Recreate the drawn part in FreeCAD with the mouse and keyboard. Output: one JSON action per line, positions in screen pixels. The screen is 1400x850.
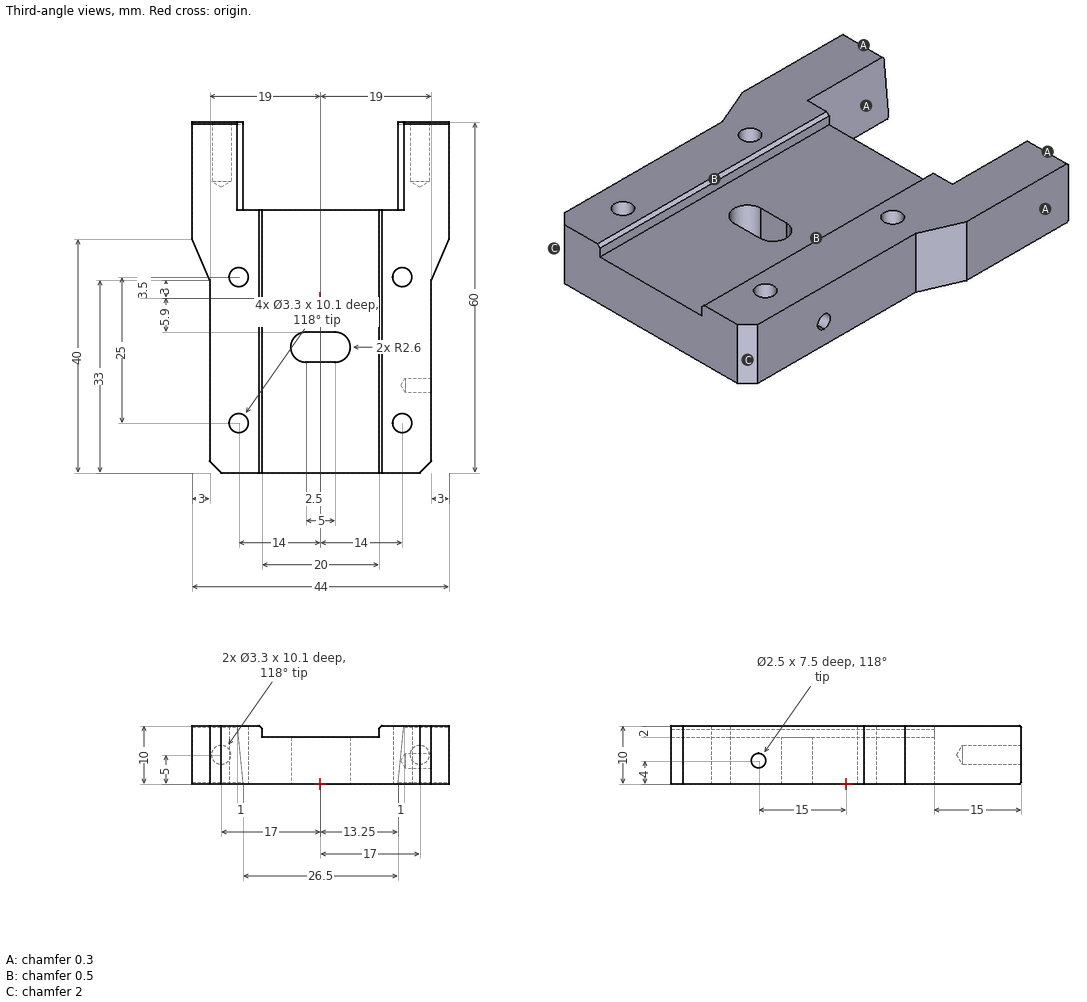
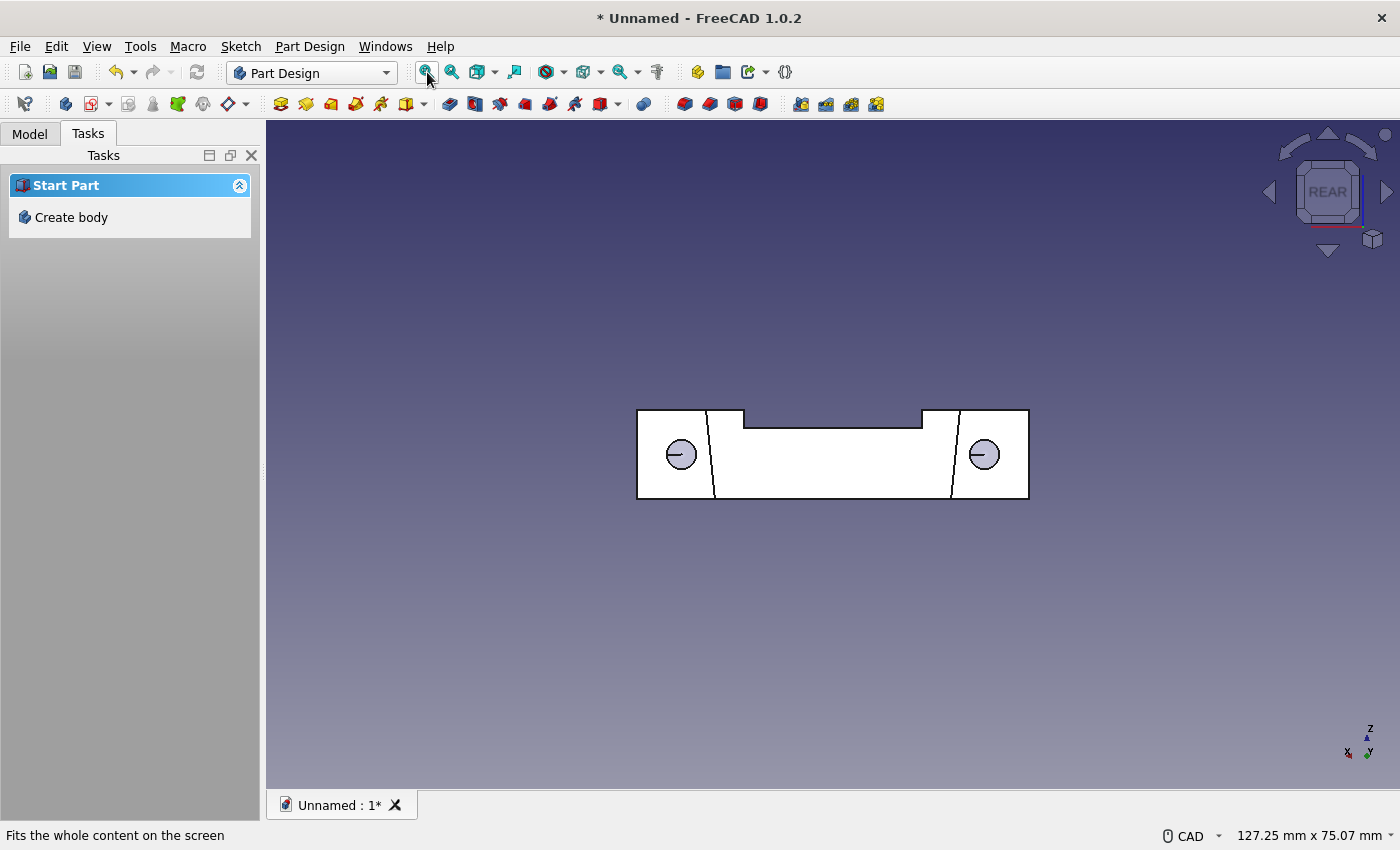
{"action": "key", "text": "0"}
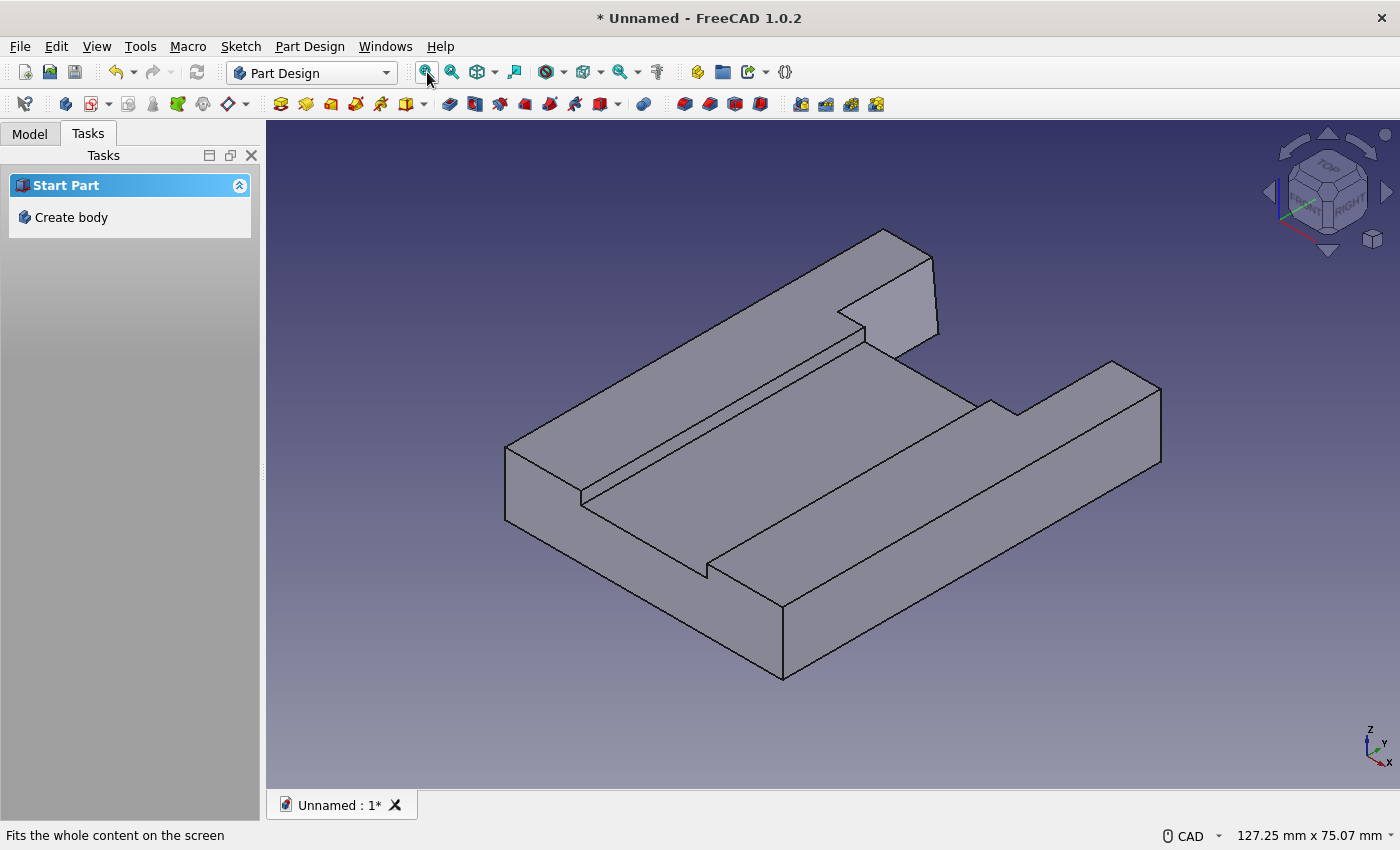
{"action": "left_click", "coordinate": [786, 328]}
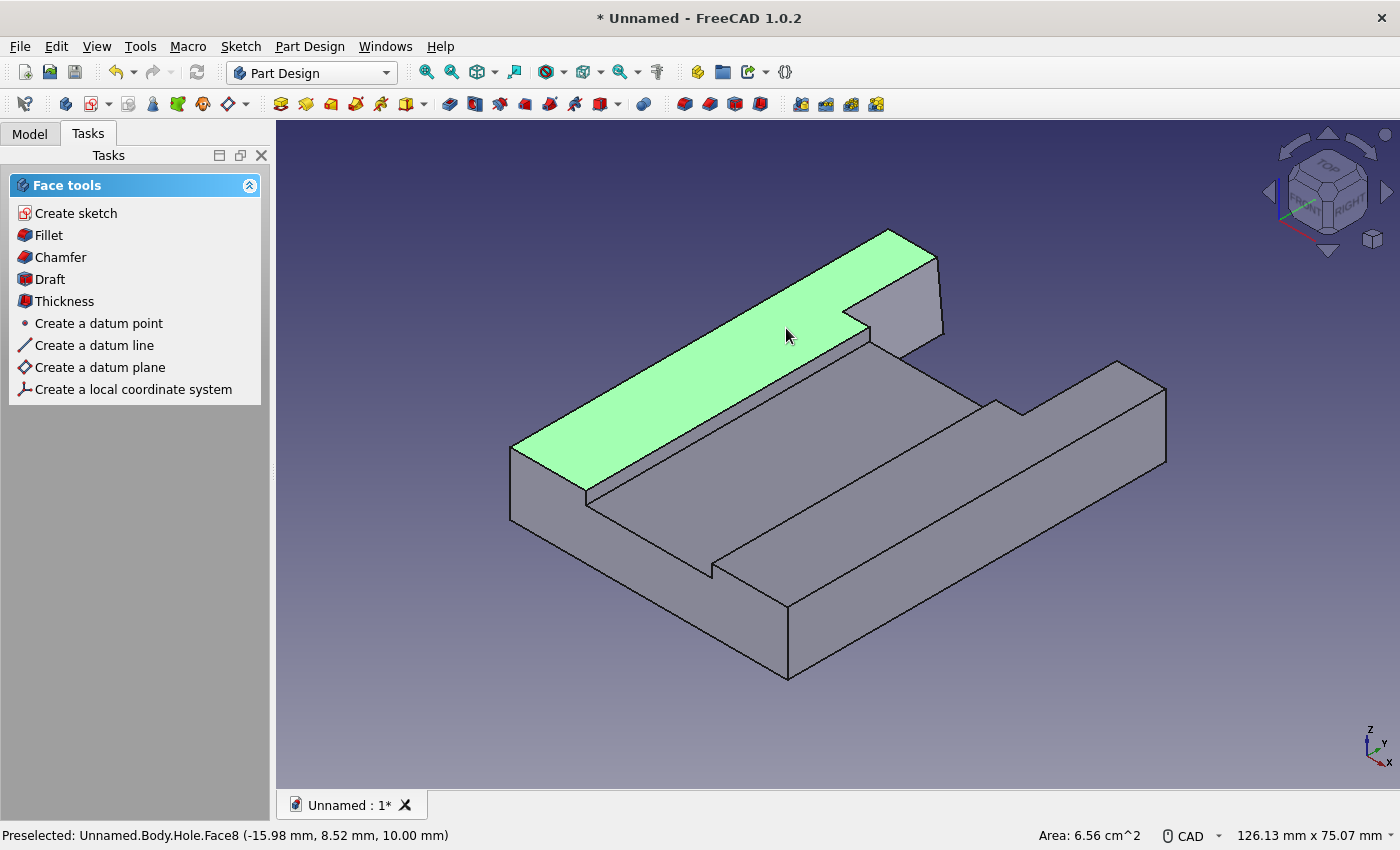
{"action": "left_click", "coordinate": [90, 104]}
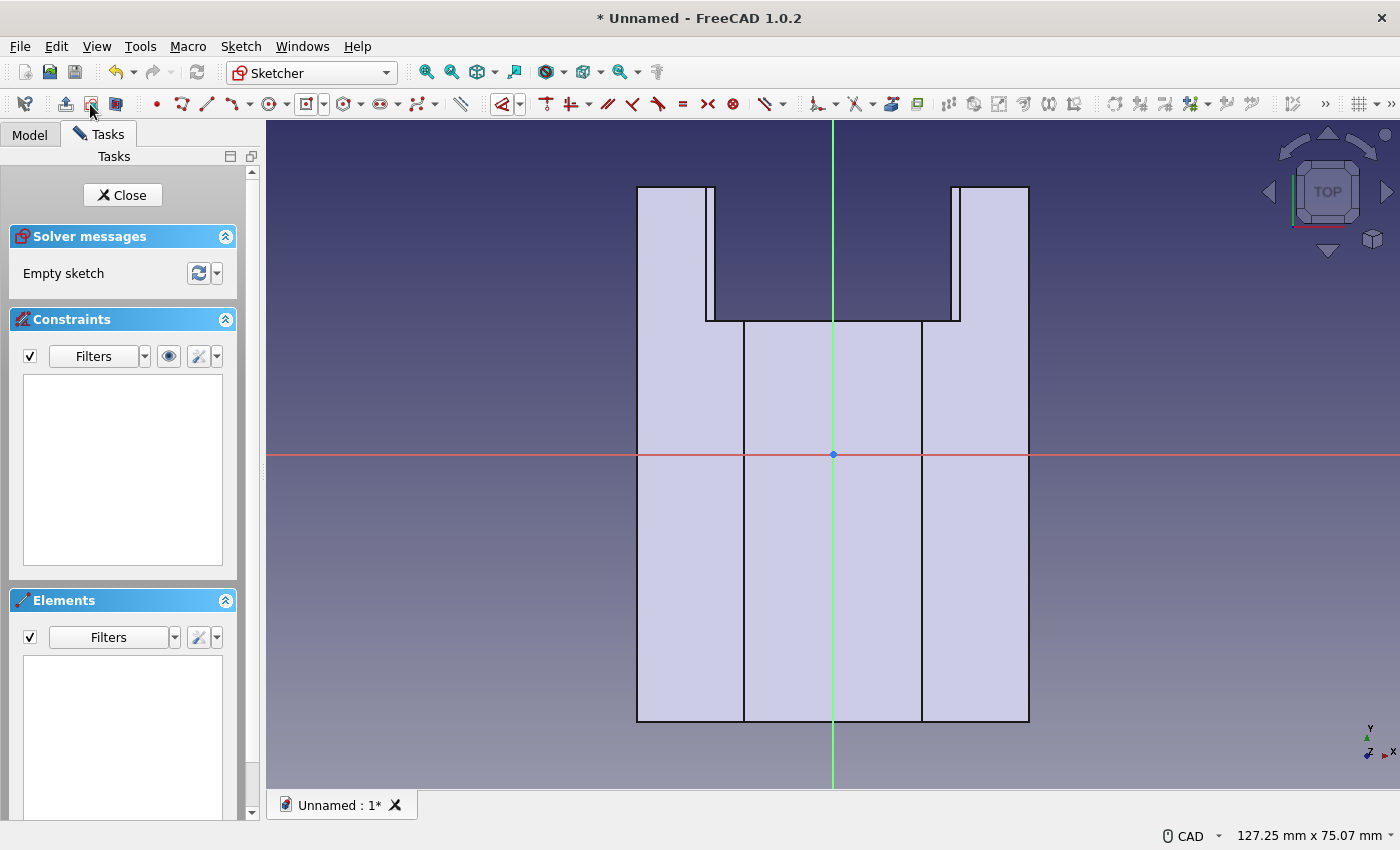
{"action": "scroll", "coordinate": [916, 632], "scroll_direction": "up", "scroll_amount": 3}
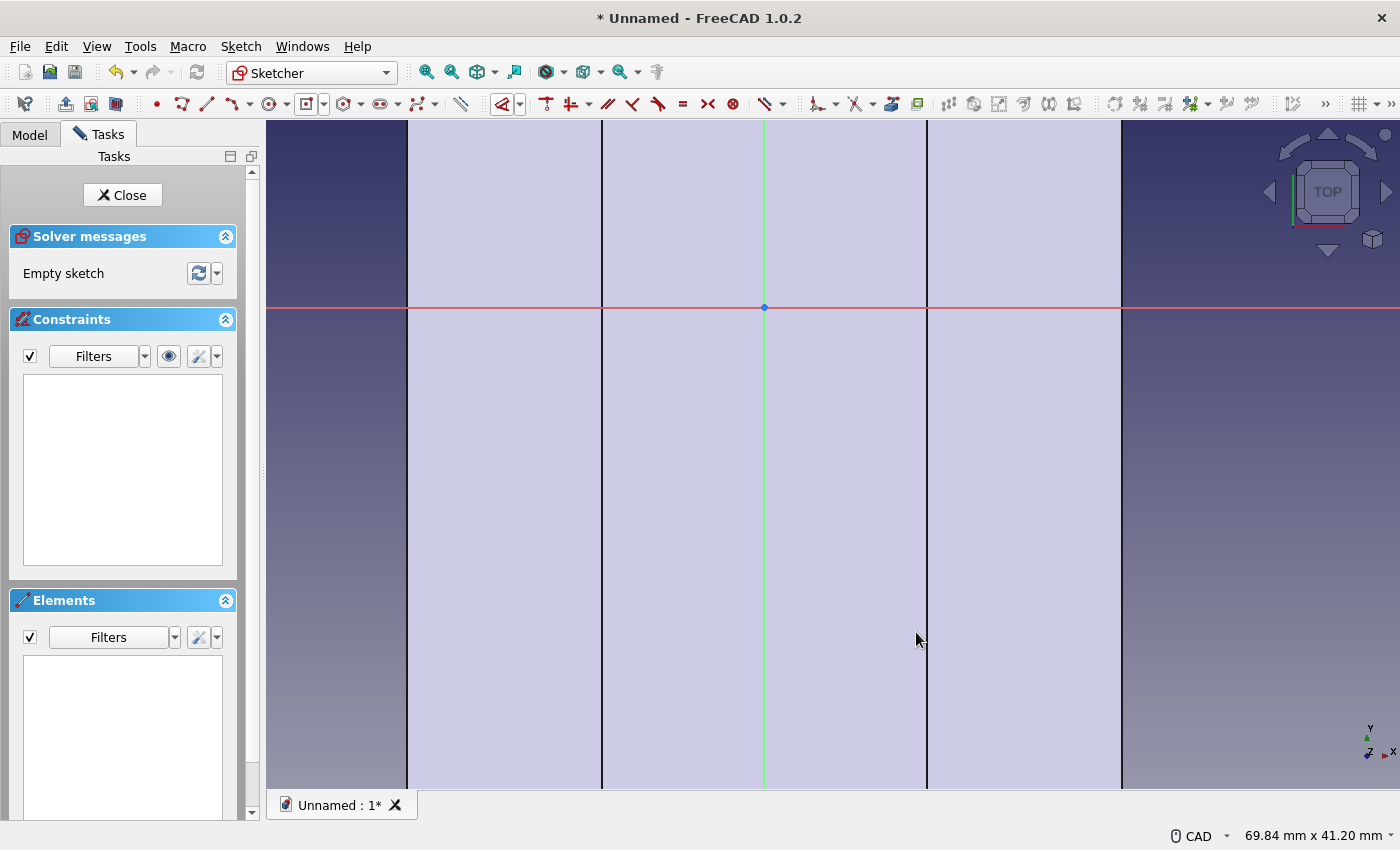
{"action": "key", "text": "g c"}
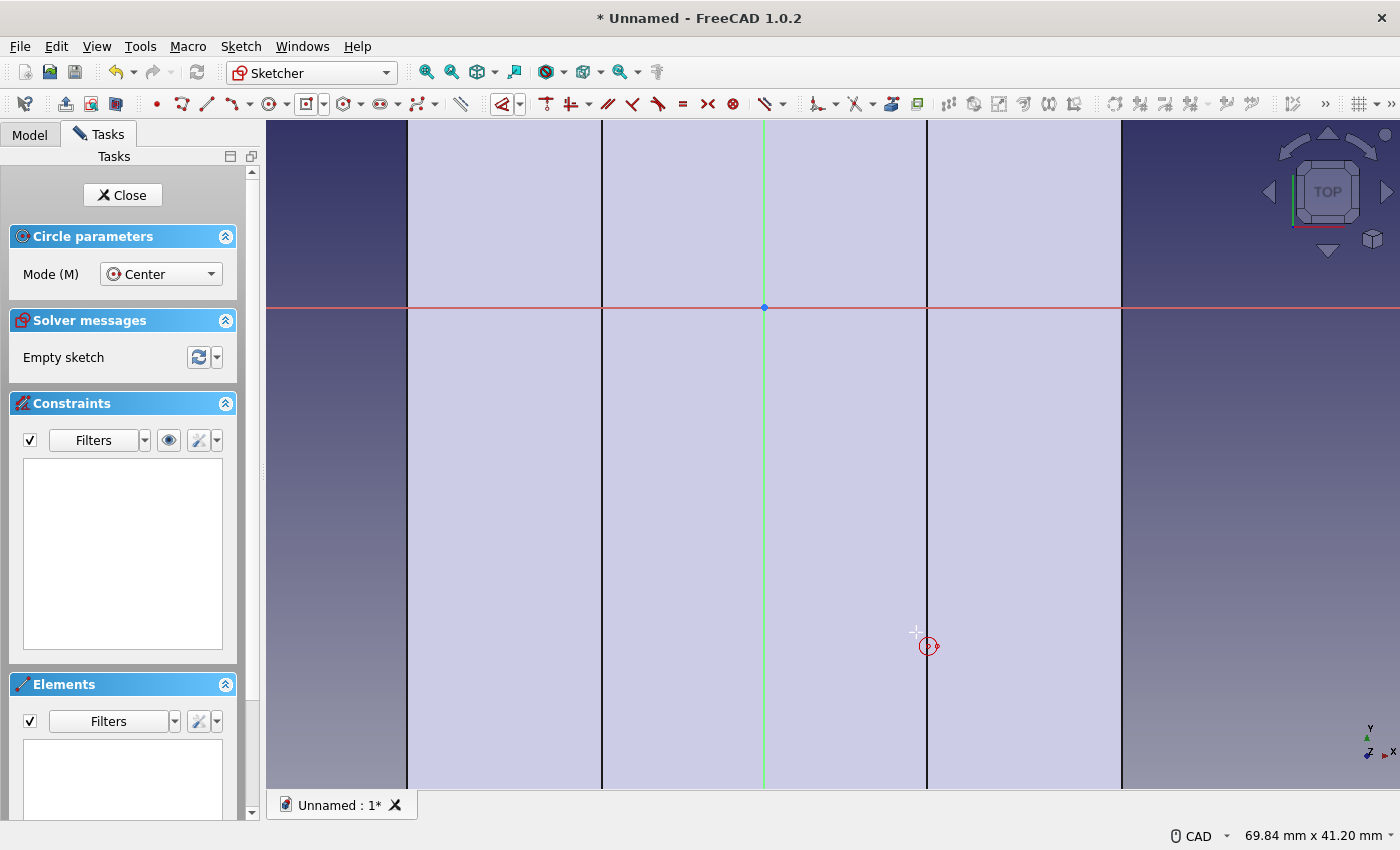
{"action": "left_click", "coordinate": [537, 657]}
{"action": "left_click", "coordinate": [556, 638]}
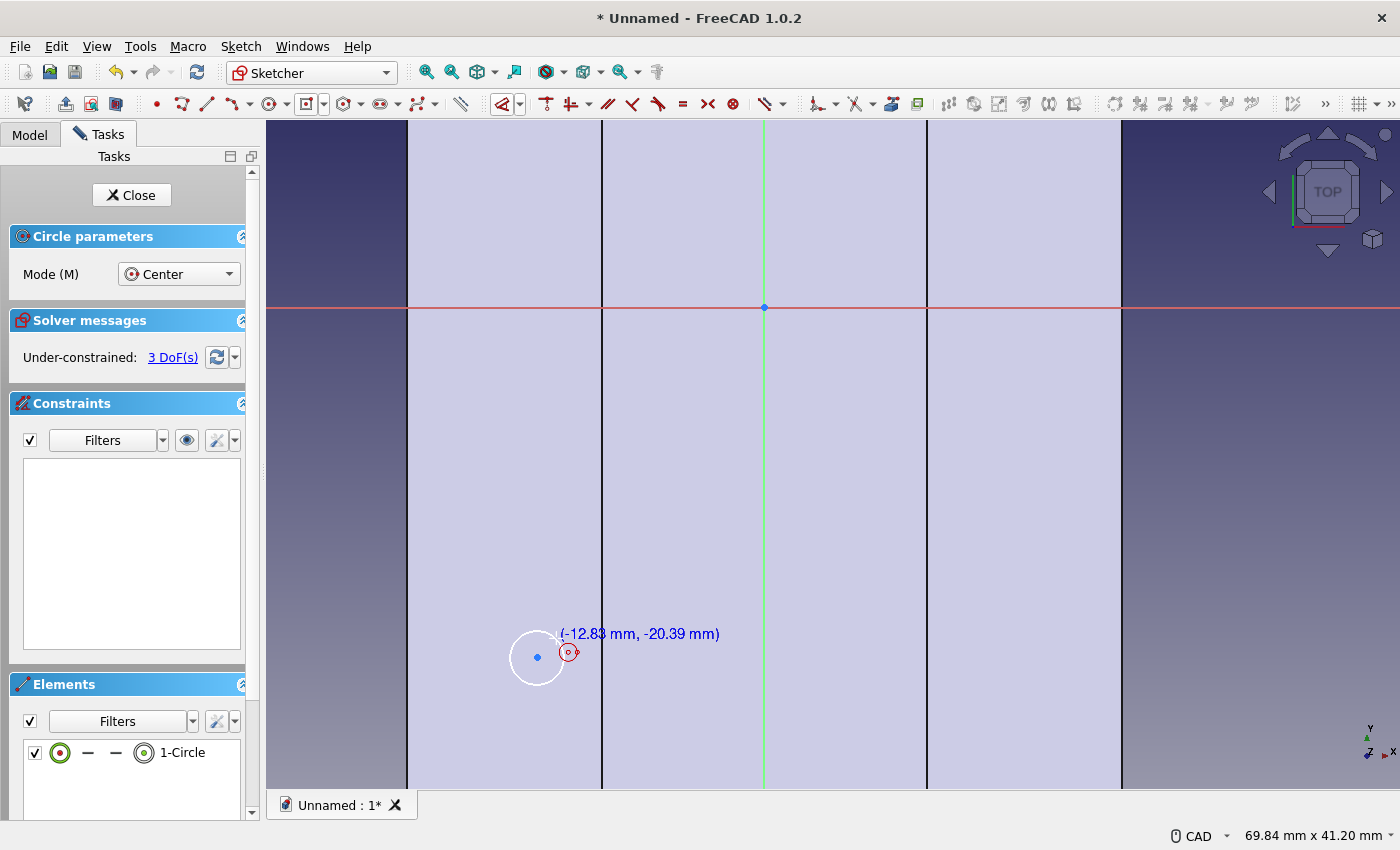
{"action": "left_click", "coordinate": [992, 657]}
{"action": "left_click", "coordinate": [1011, 638]}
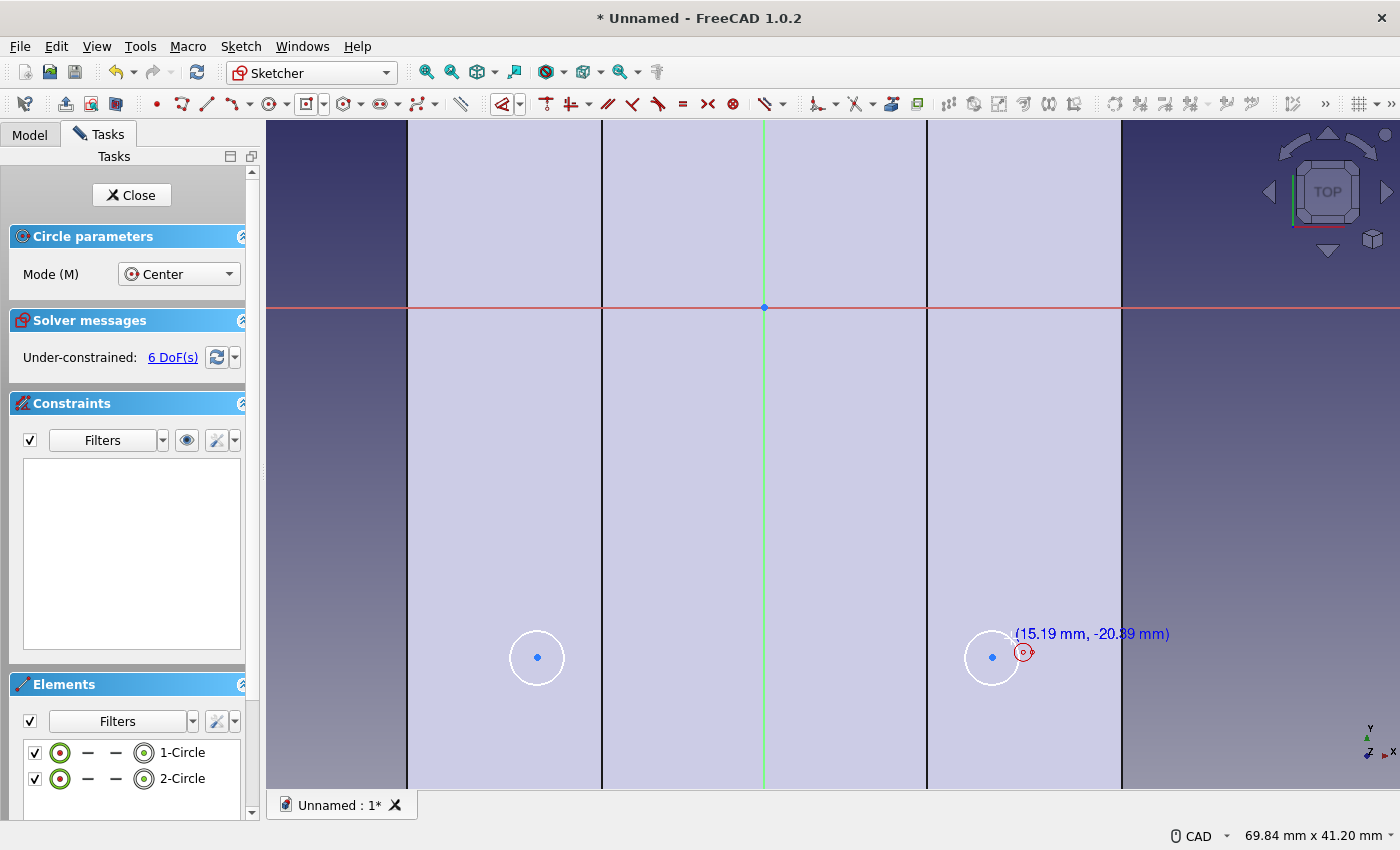
{"action": "left_click", "coordinate": [537, 251]}
{"action": "left_click", "coordinate": [556, 232]}